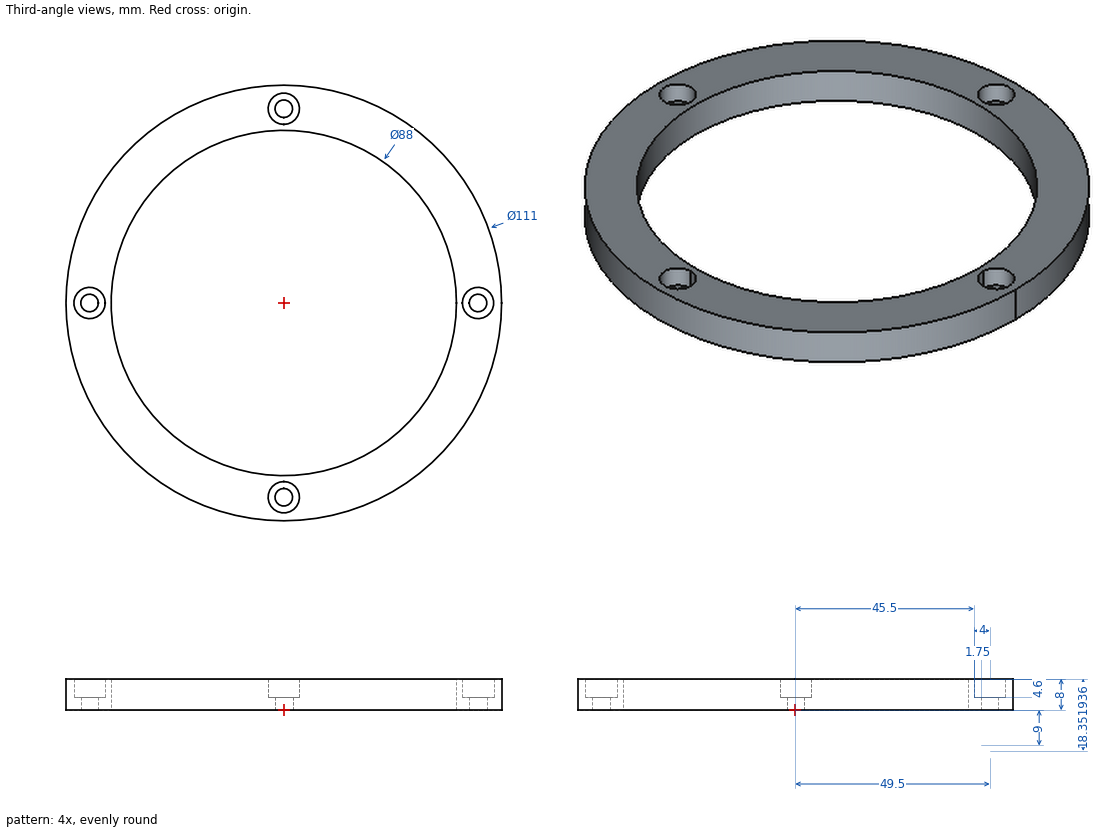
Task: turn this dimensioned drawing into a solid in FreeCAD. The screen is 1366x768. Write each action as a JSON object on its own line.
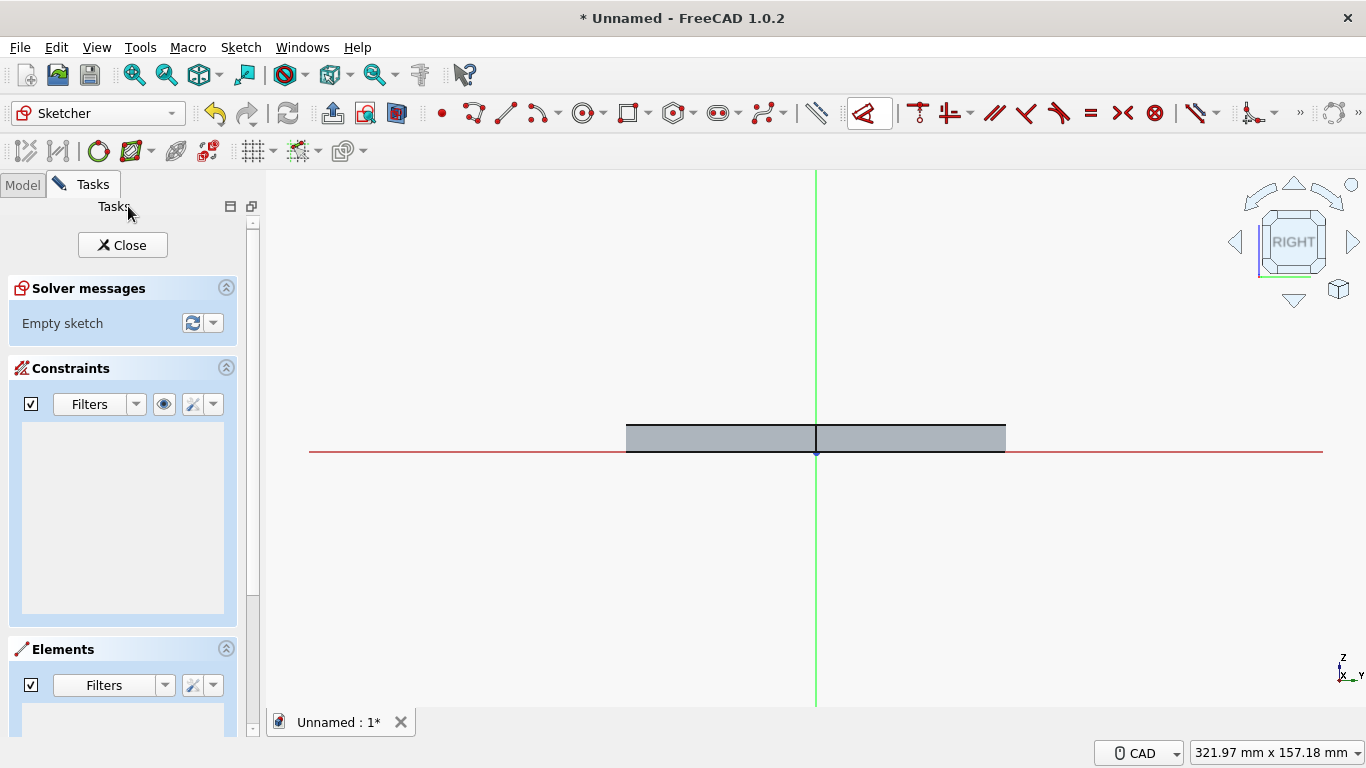
{"action": "left_click", "coordinate": [398, 114]}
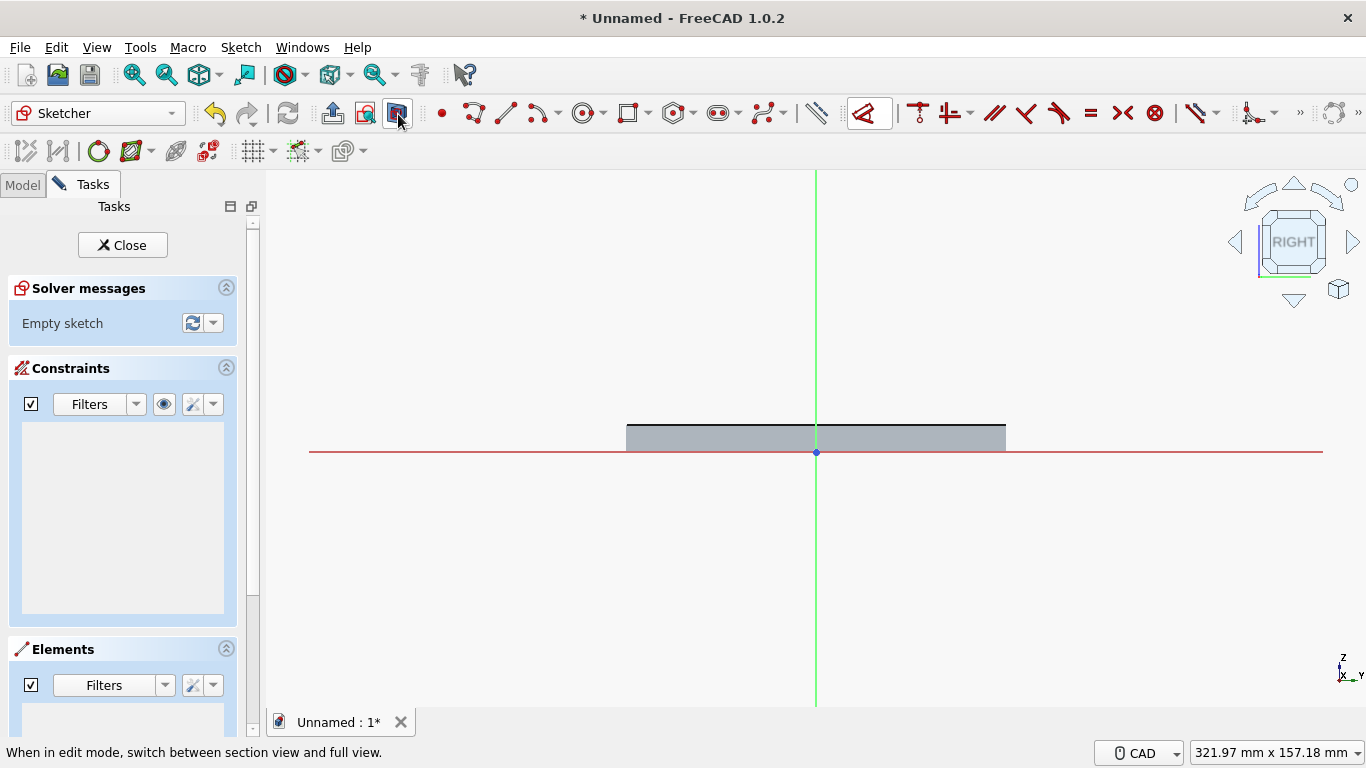
{"action": "scroll", "coordinate": [951, 479], "scroll_direction": "up", "scroll_amount": 7}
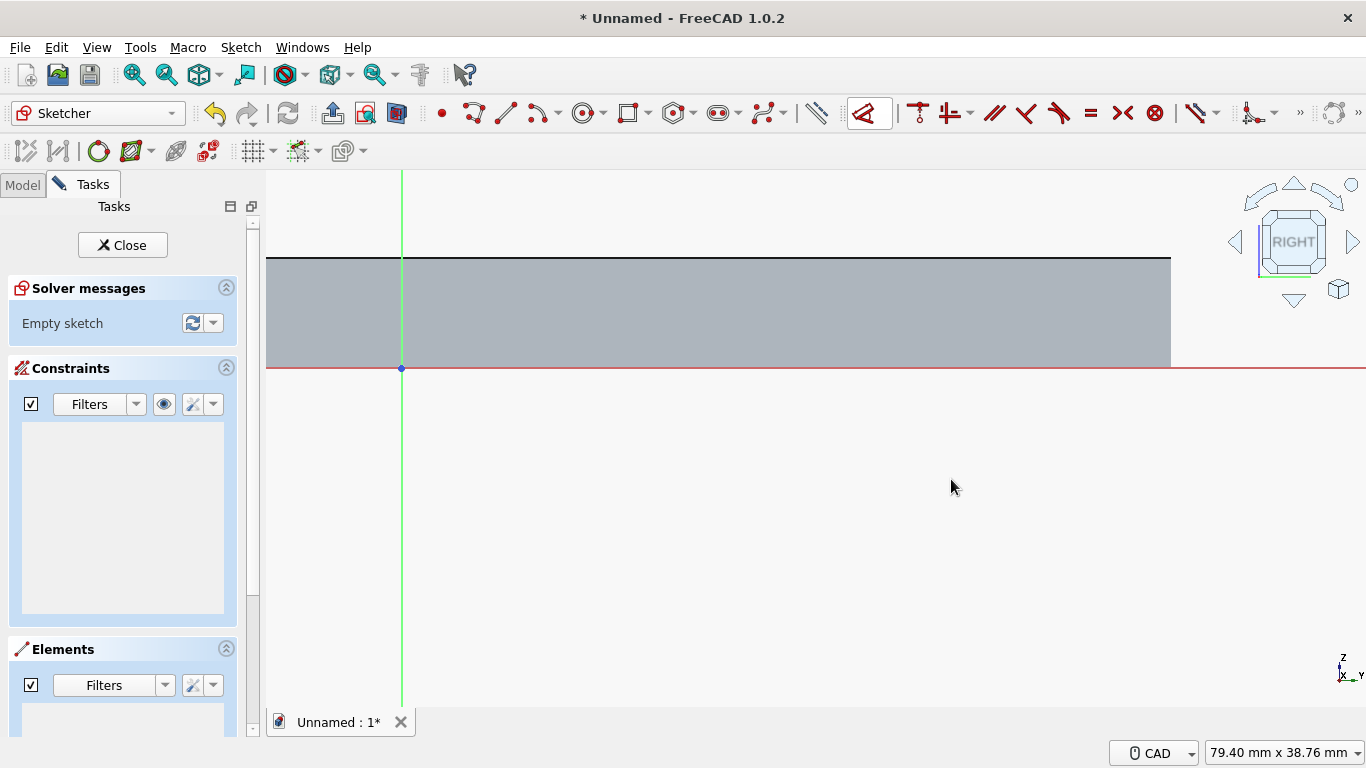
{"action": "key", "text": "g m"}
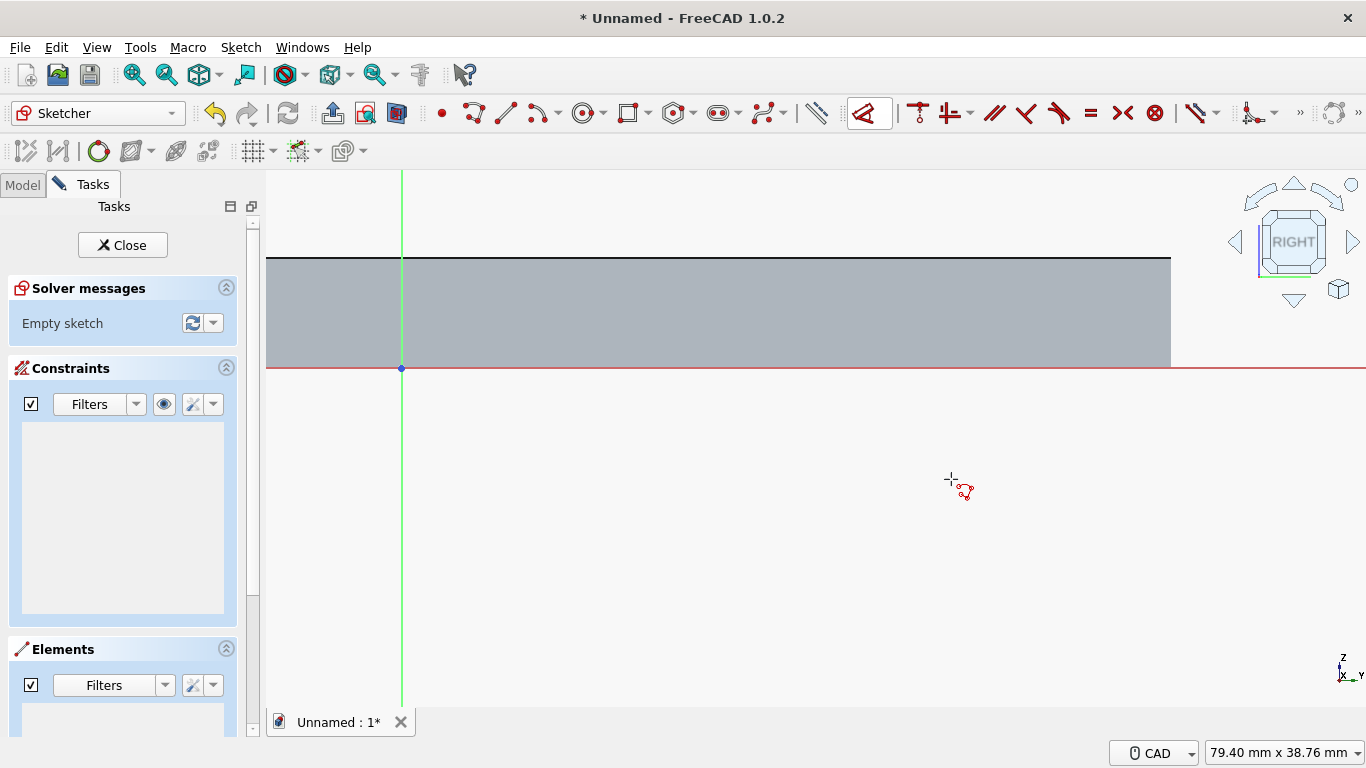
{"action": "left_click", "coordinate": [1032, 321]}
{"action": "left_click", "coordinate": [1056, 321]}
{"action": "left_click", "coordinate": [1056, 493]}
{"action": "left_click", "coordinate": [1087, 512]}
{"action": "left_click", "coordinate": [1087, 258]}
{"action": "left_click", "coordinate": [1032, 258]}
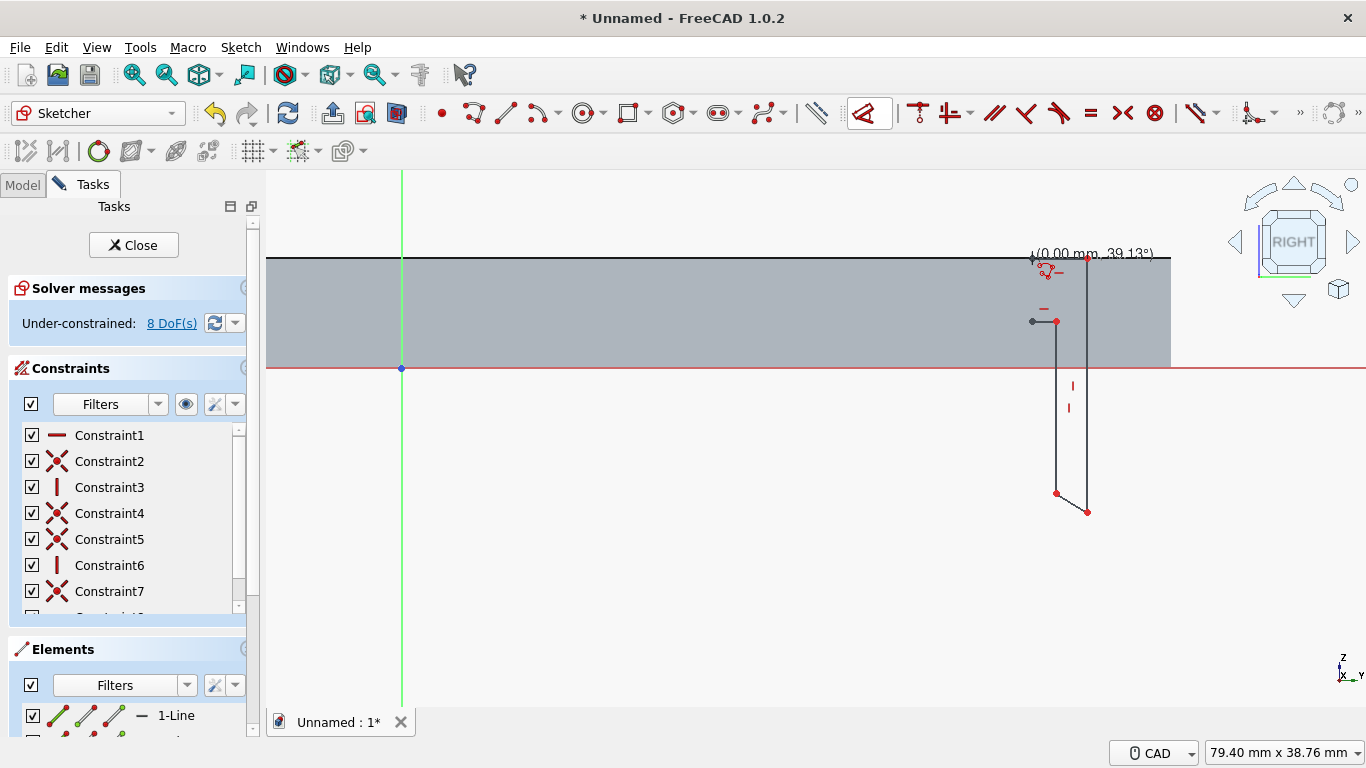
{"action": "scroll", "coordinate": [1032, 321], "scroll_direction": "up", "scroll_amount": 2}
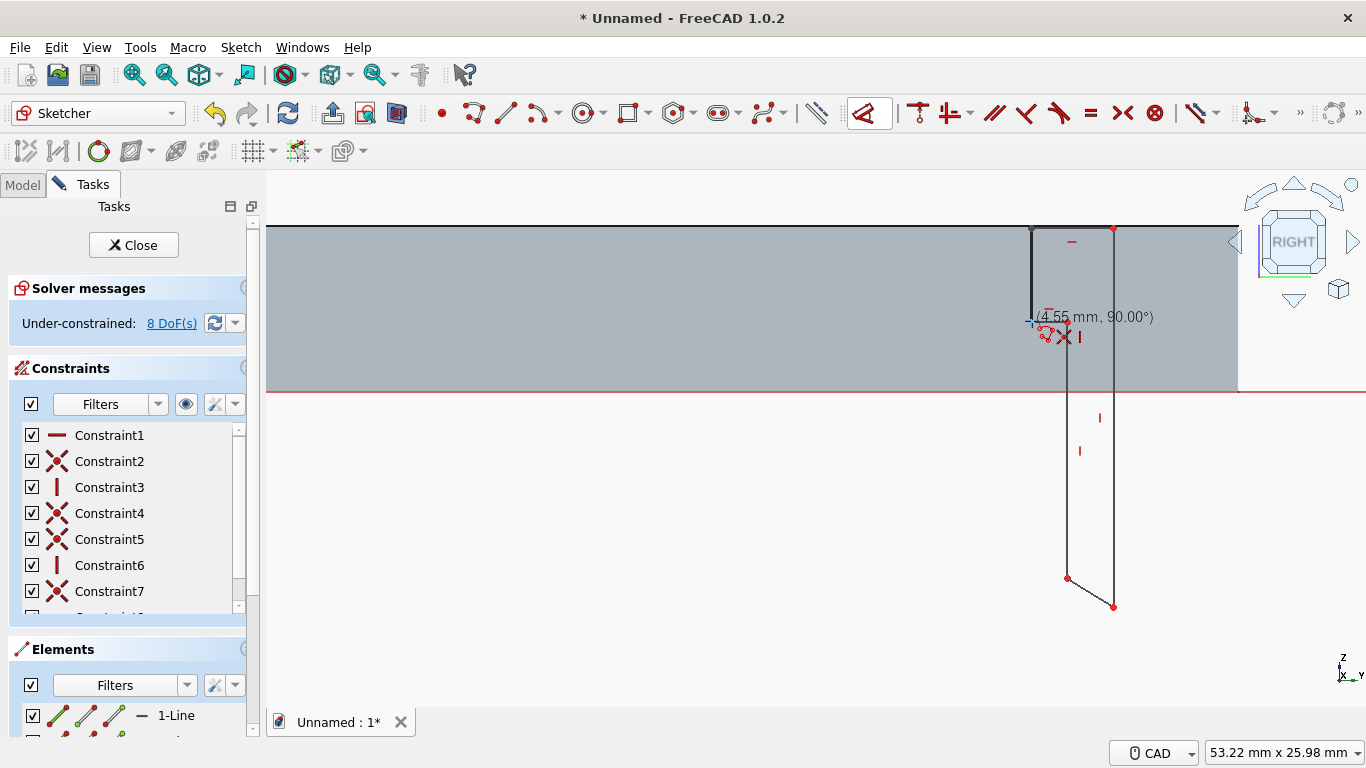
{"action": "left_click", "coordinate": [1032, 322]}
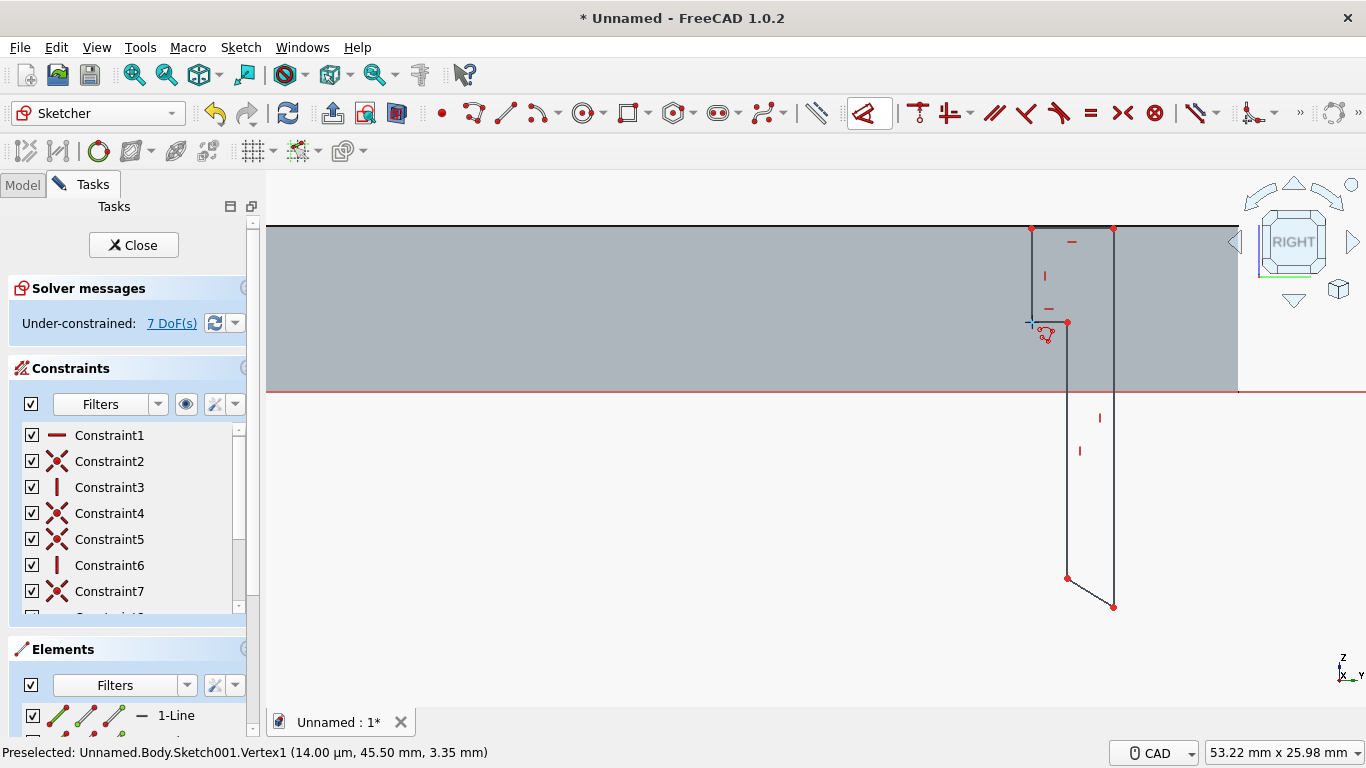
{"action": "key", "text": "g l"}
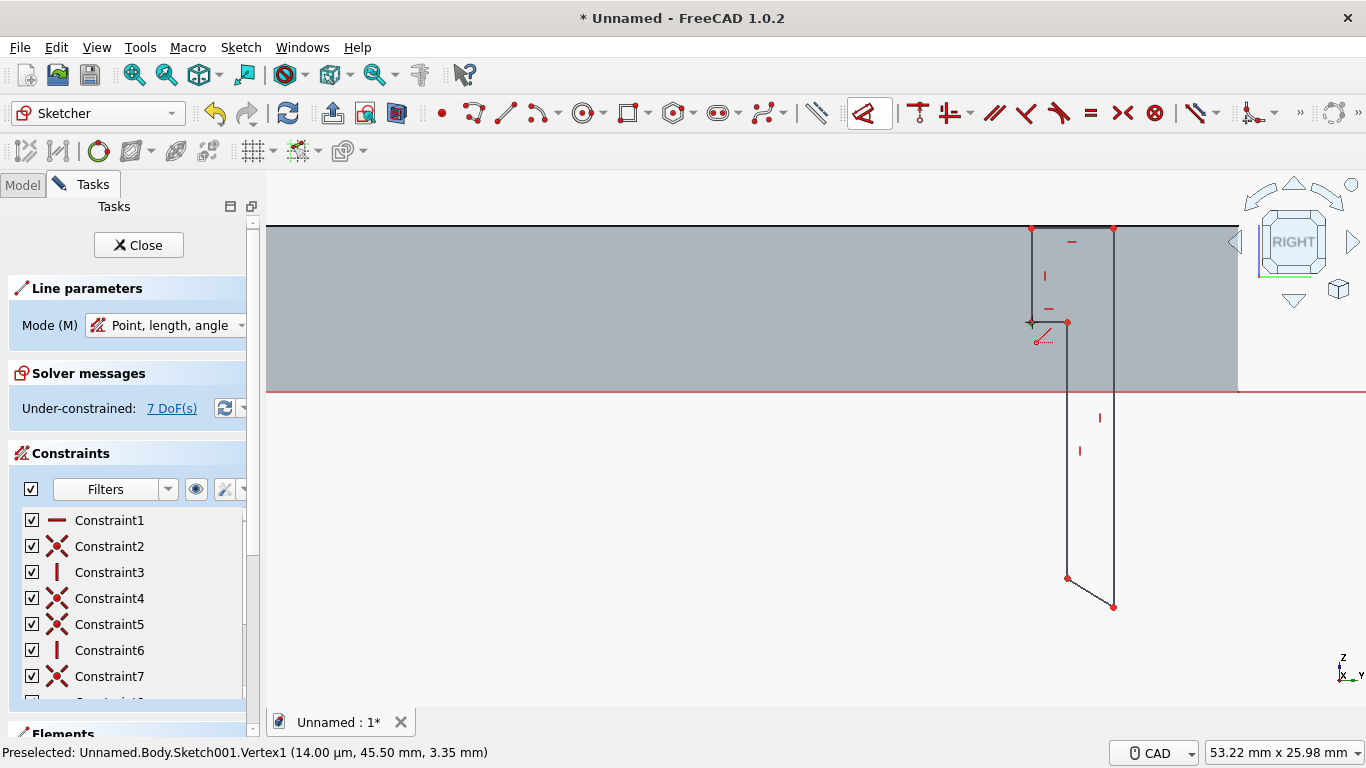
{"action": "left_click", "coordinate": [1114, 643]}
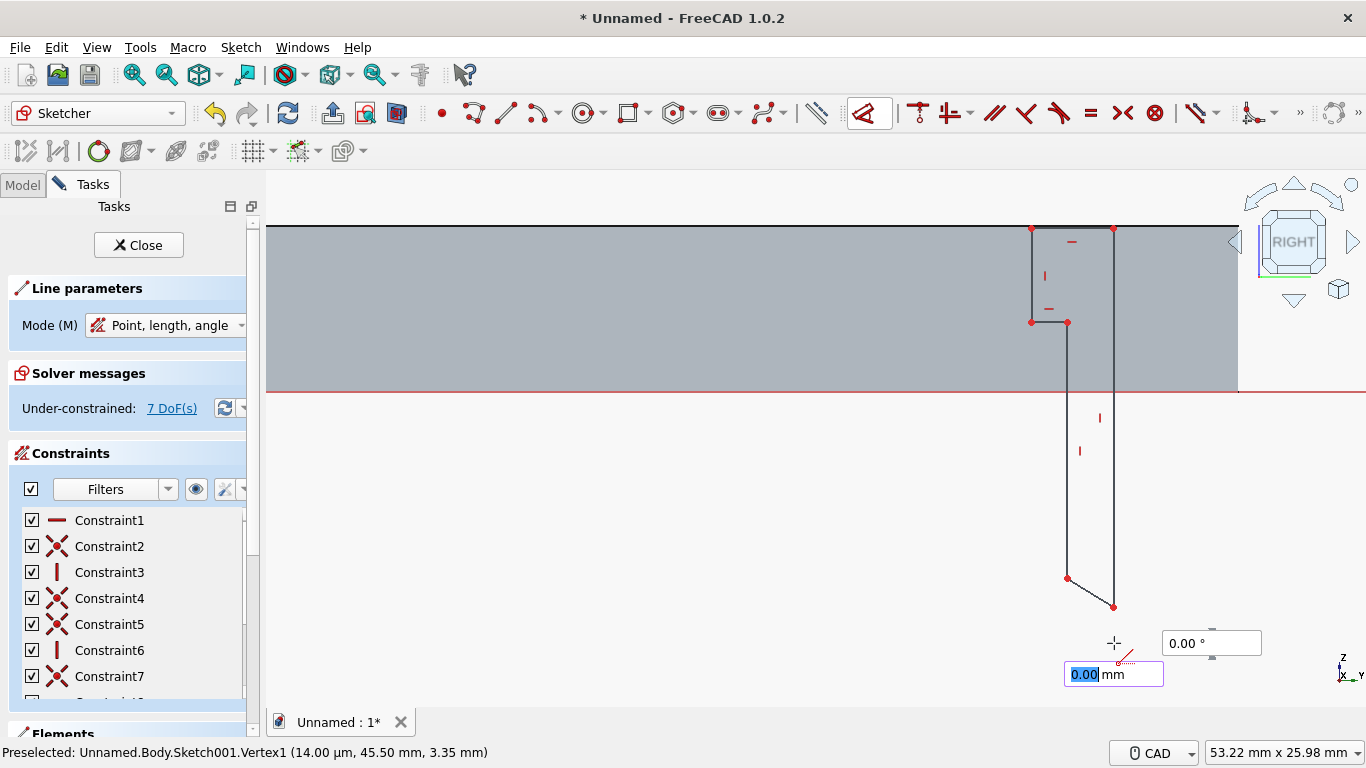
{"action": "scroll", "coordinate": [1042, 330], "scroll_direction": "down", "scroll_amount": 2}